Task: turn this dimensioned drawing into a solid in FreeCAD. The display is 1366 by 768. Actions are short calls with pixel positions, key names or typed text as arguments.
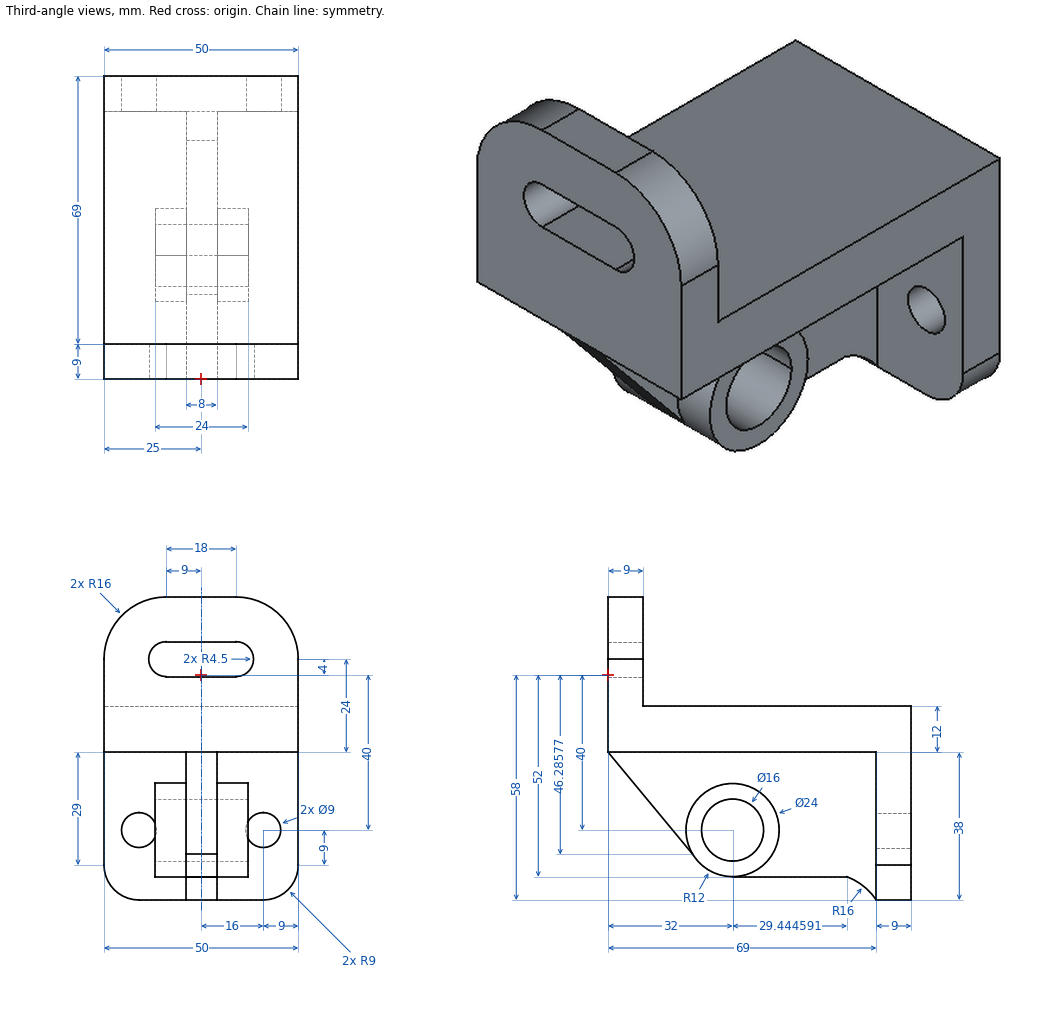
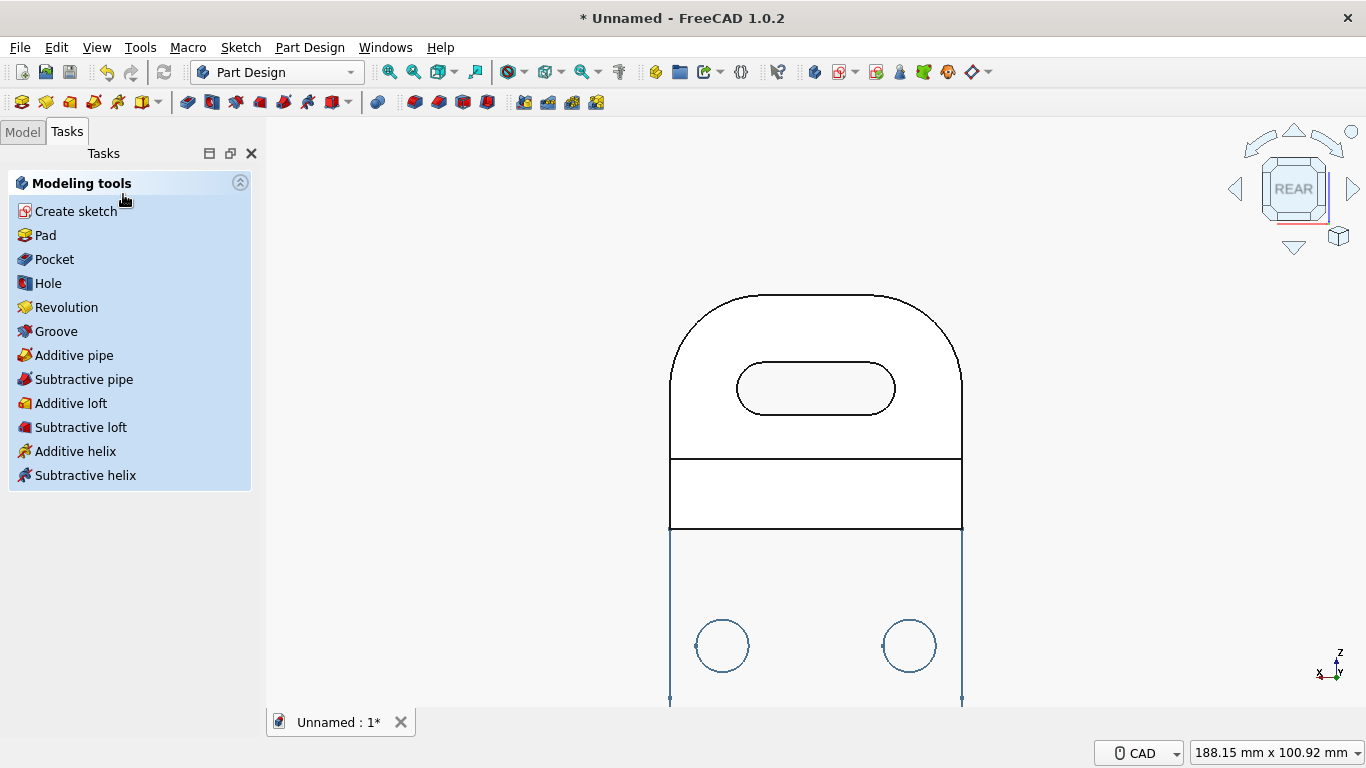
click(22, 102)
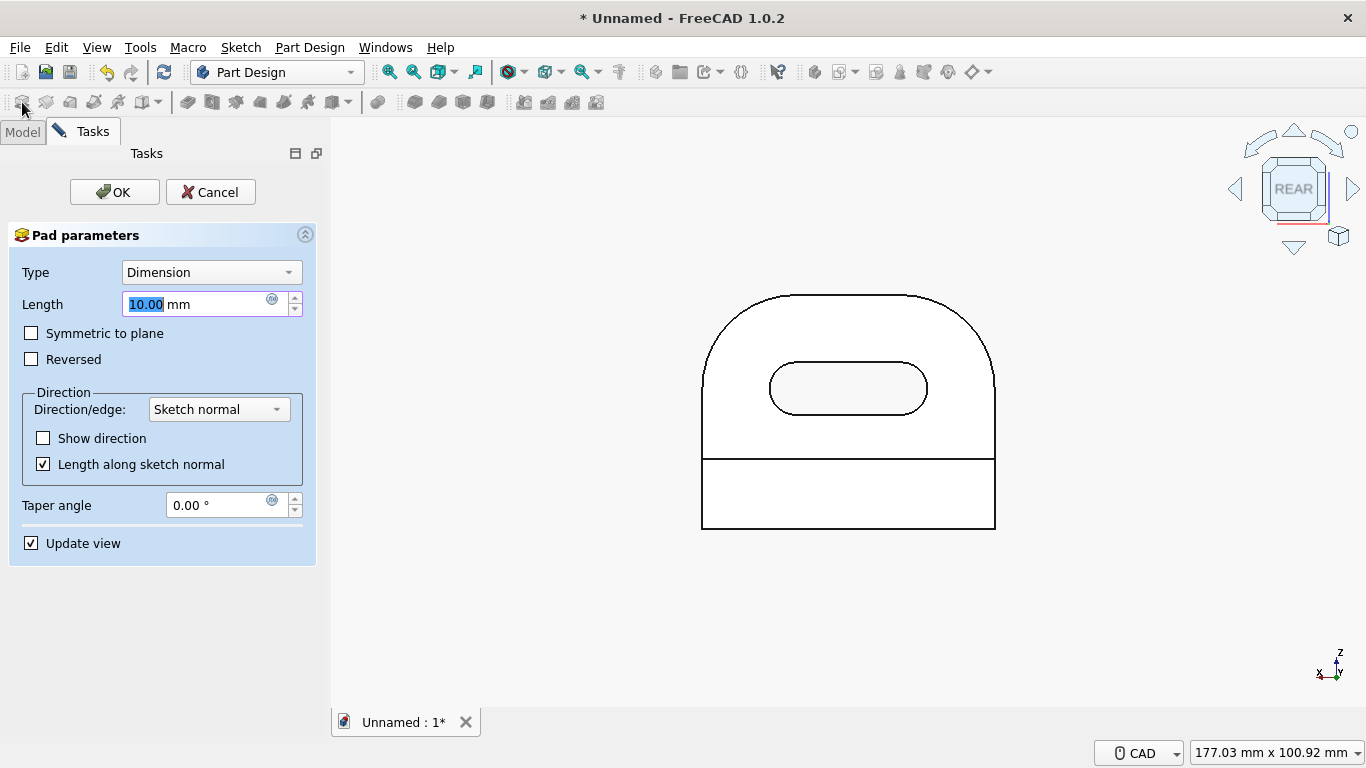
text(9)
key(Tab)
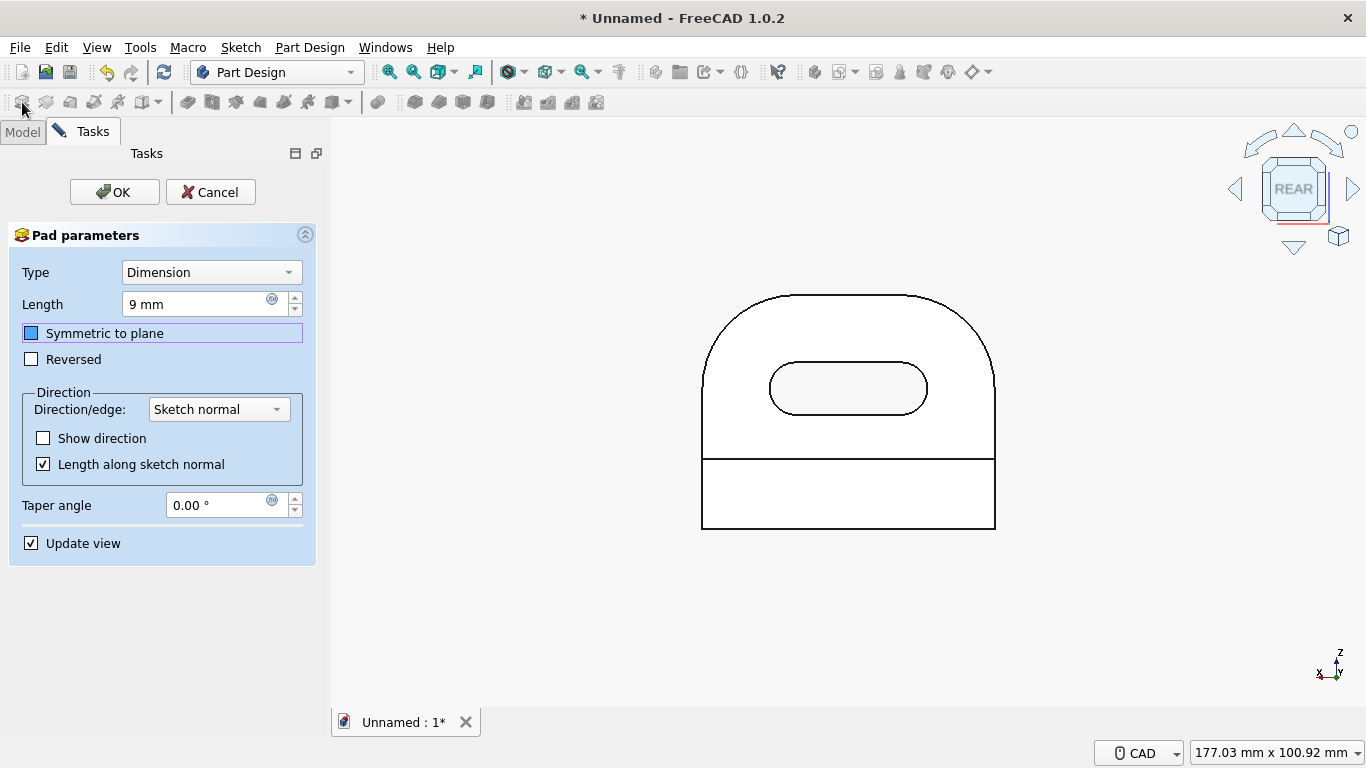
click(30, 359)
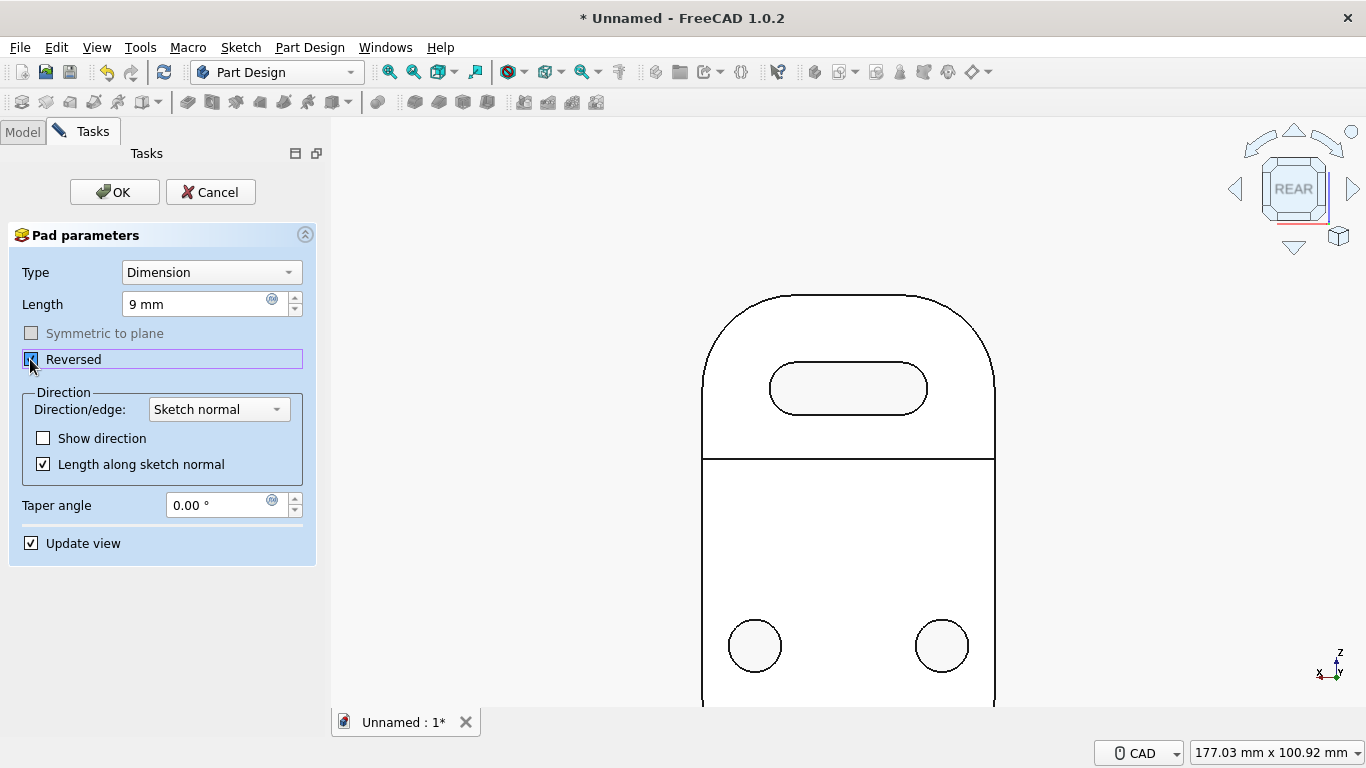
click(115, 192)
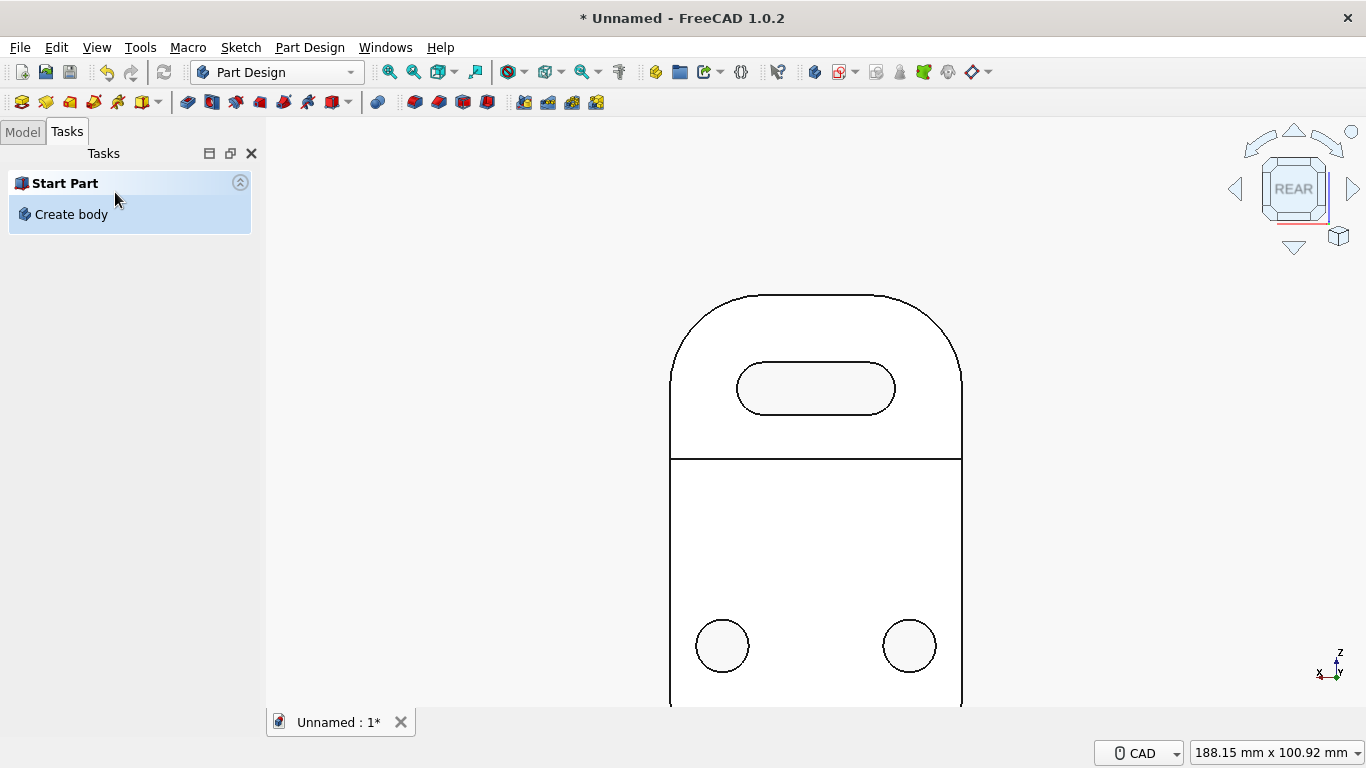
click(390, 72)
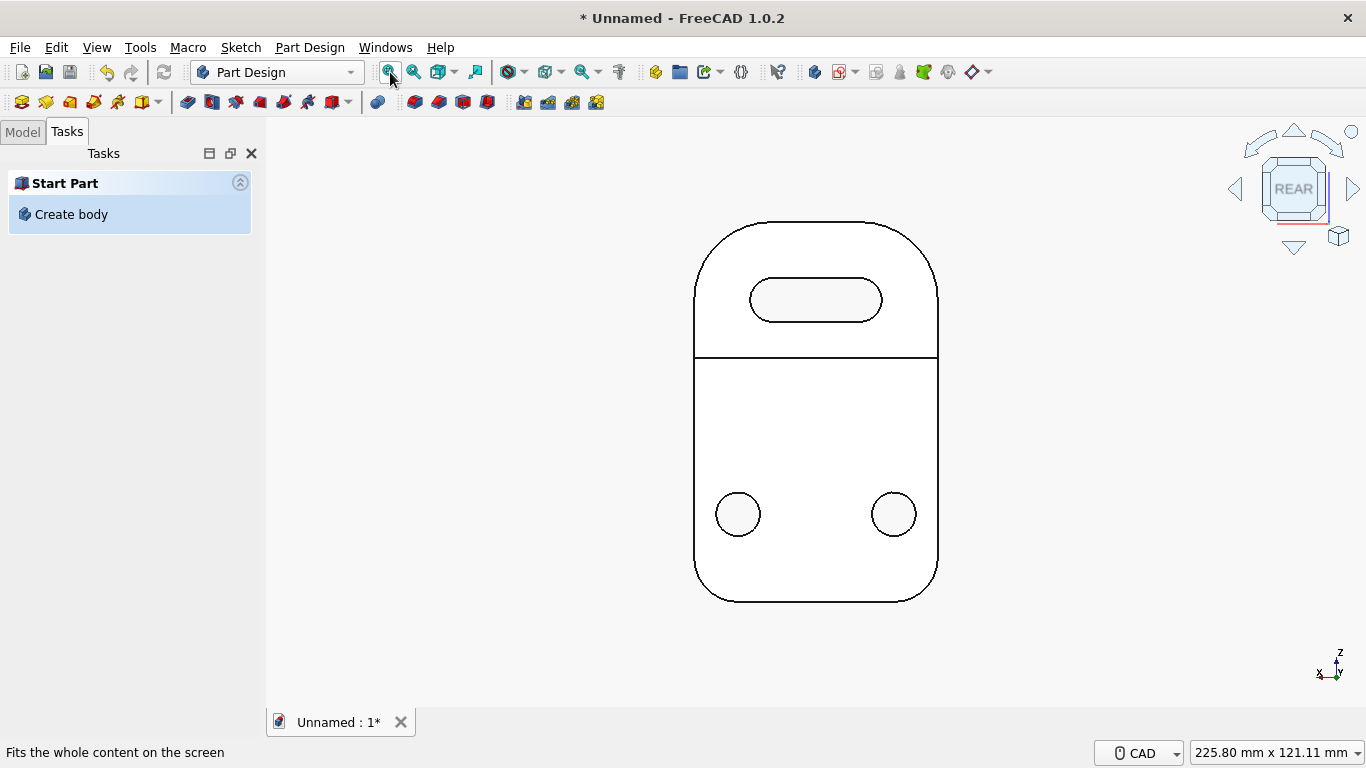
click(816, 72)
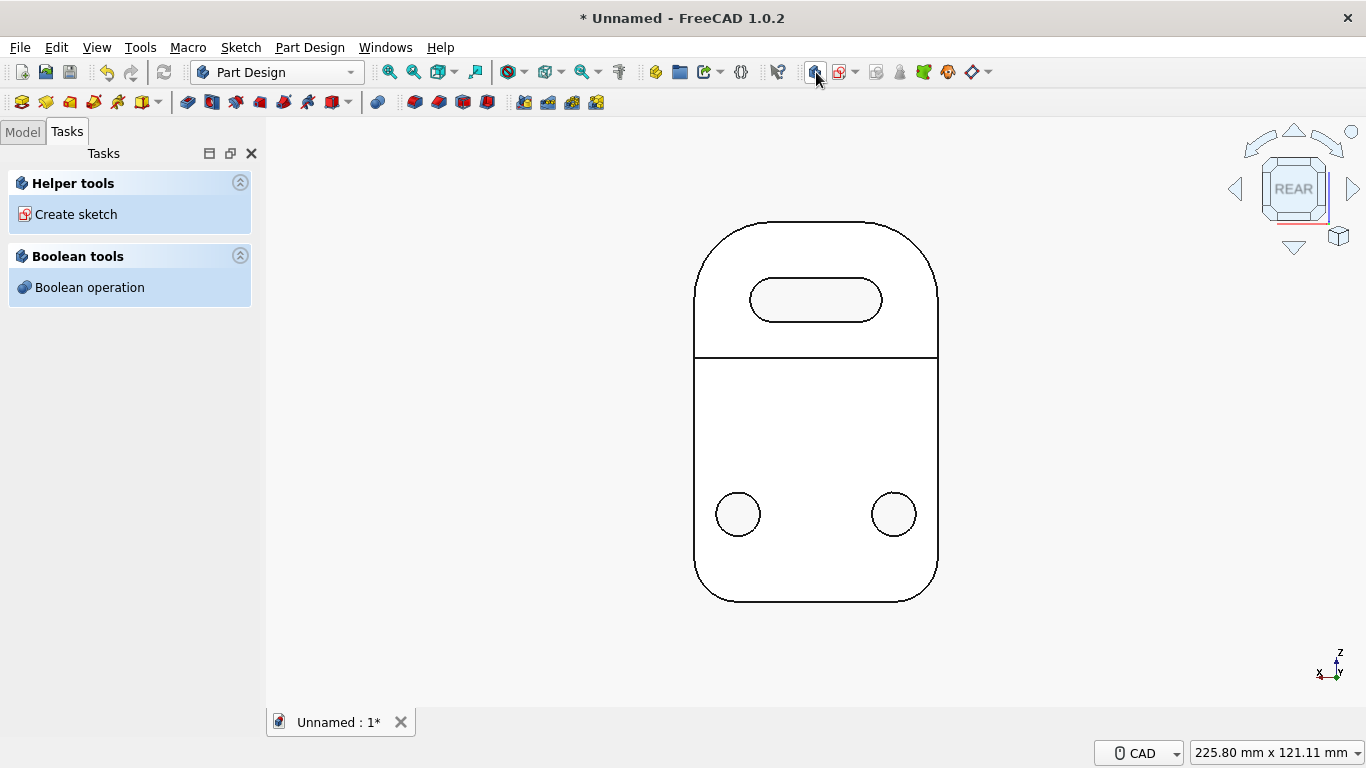
click(306, 667)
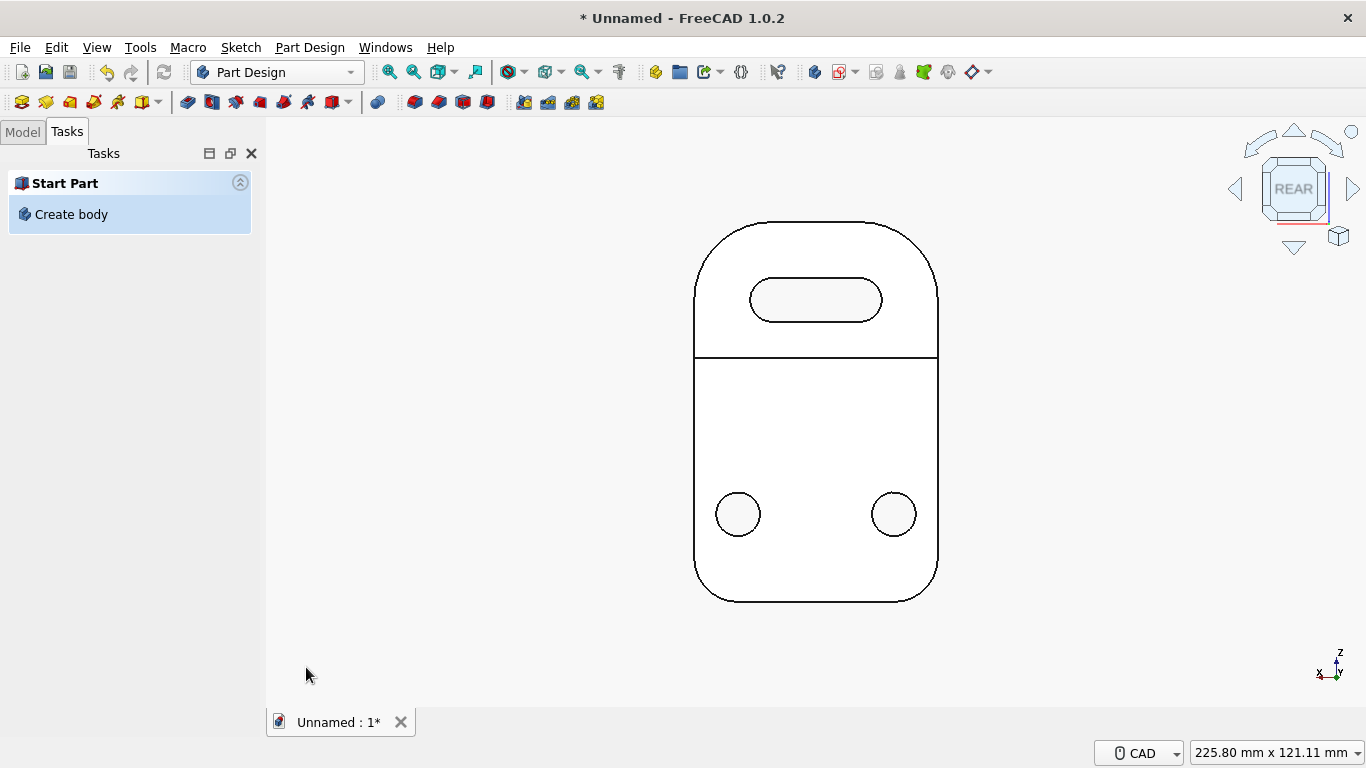
click(840, 72)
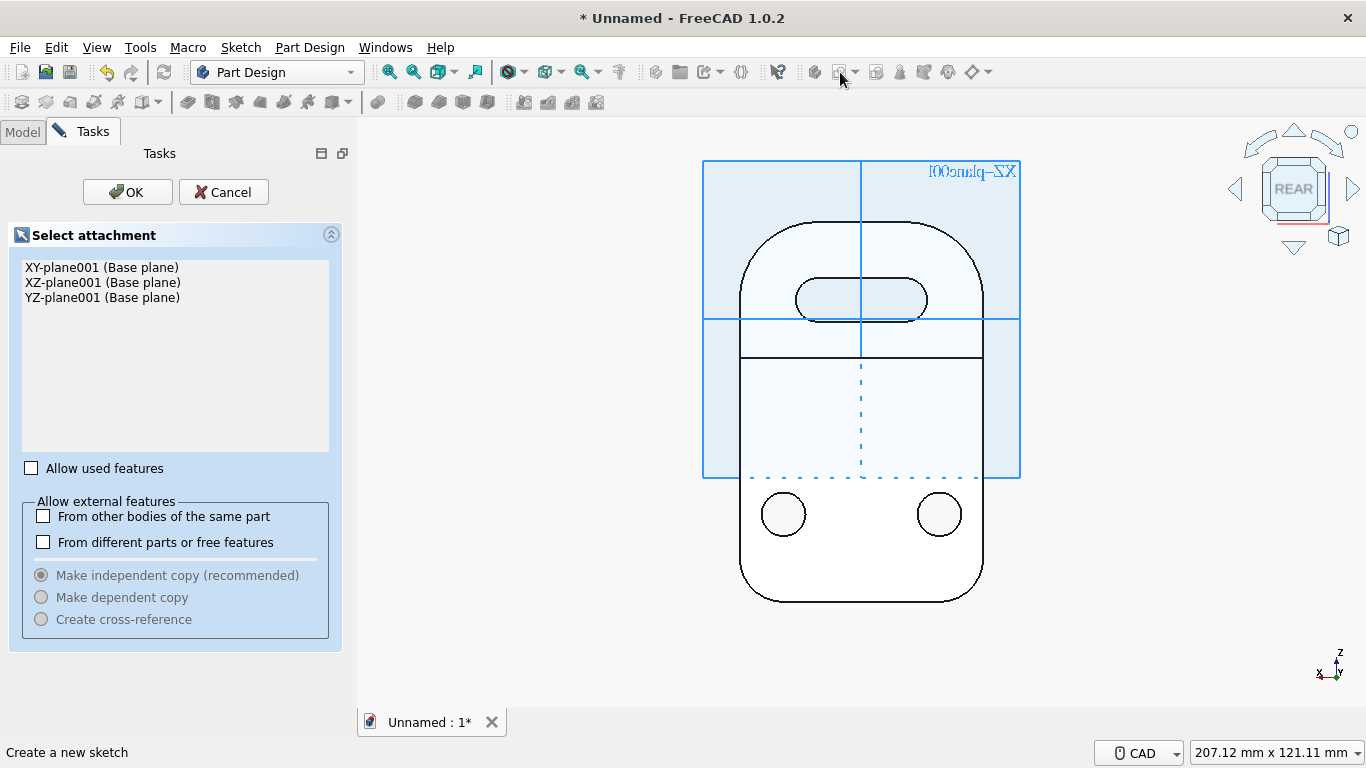
click(82, 298)